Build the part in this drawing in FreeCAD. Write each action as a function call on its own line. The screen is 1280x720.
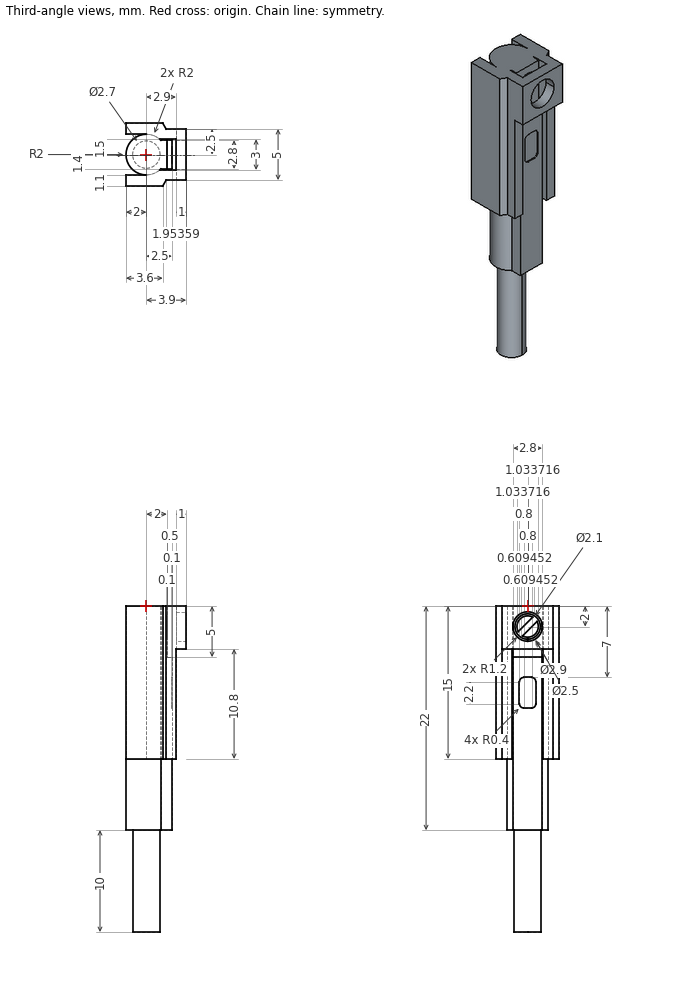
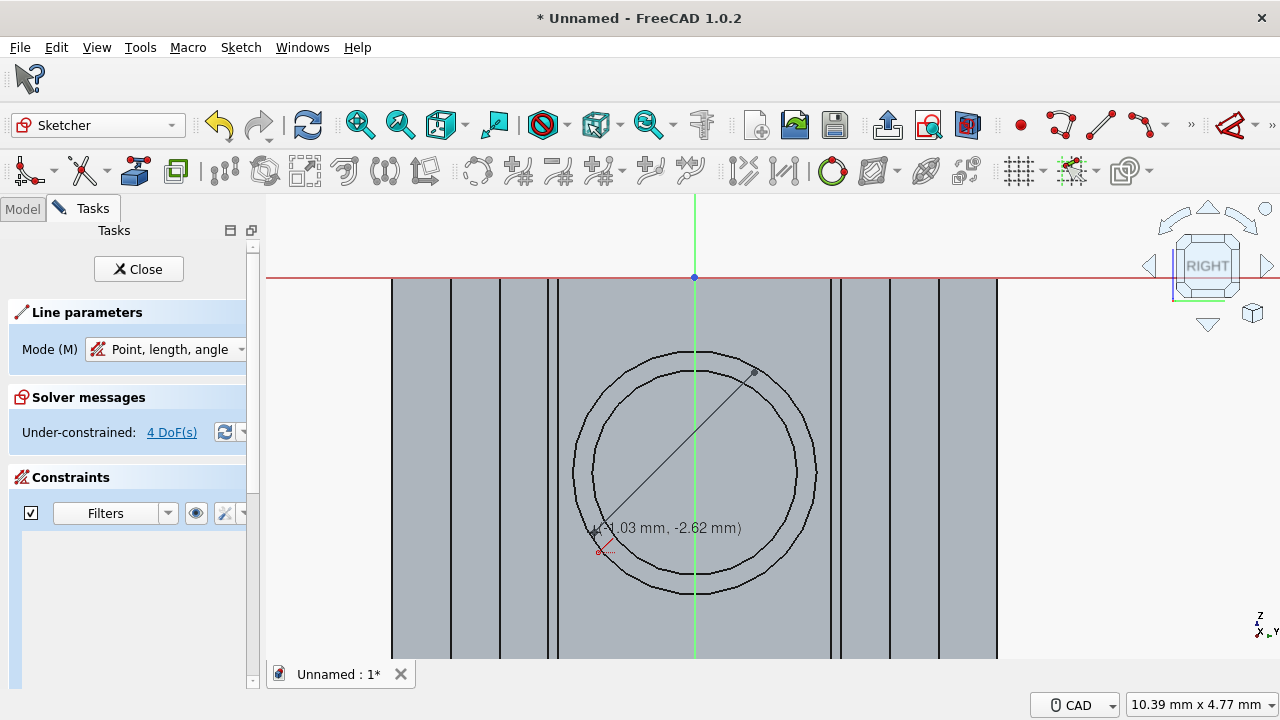
click(635, 574)
click(796, 413)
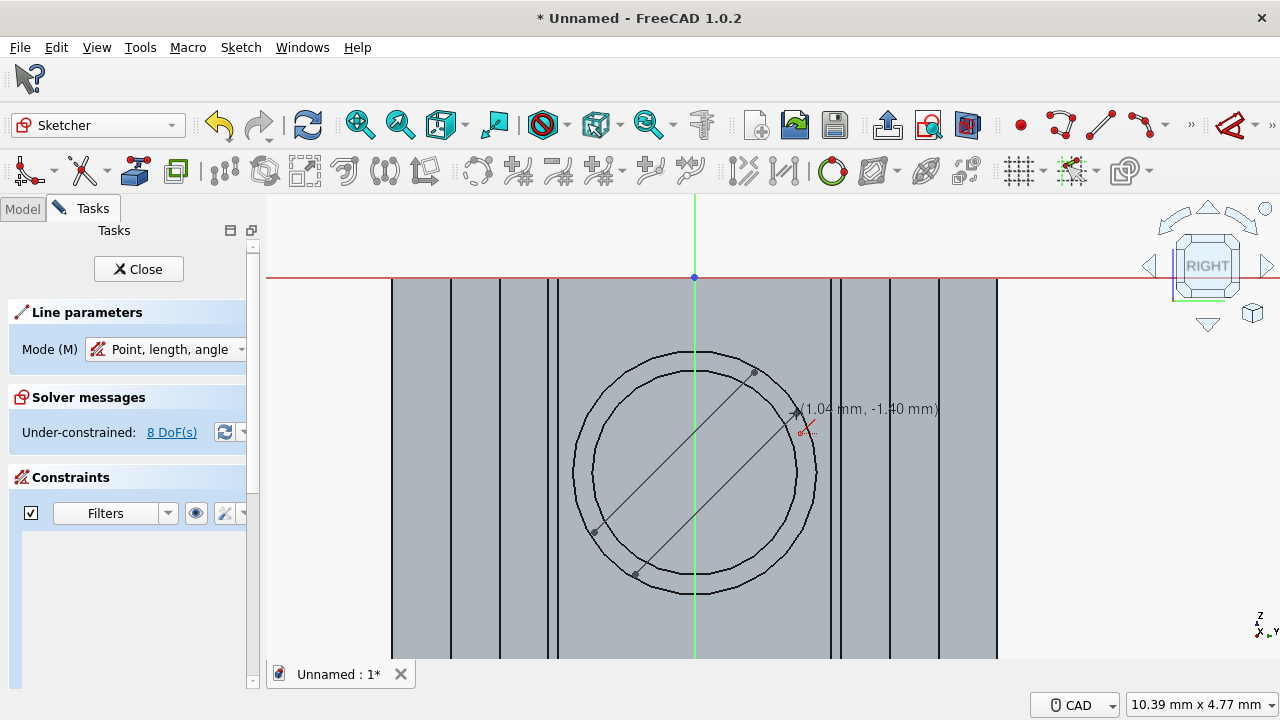
click(1142, 126)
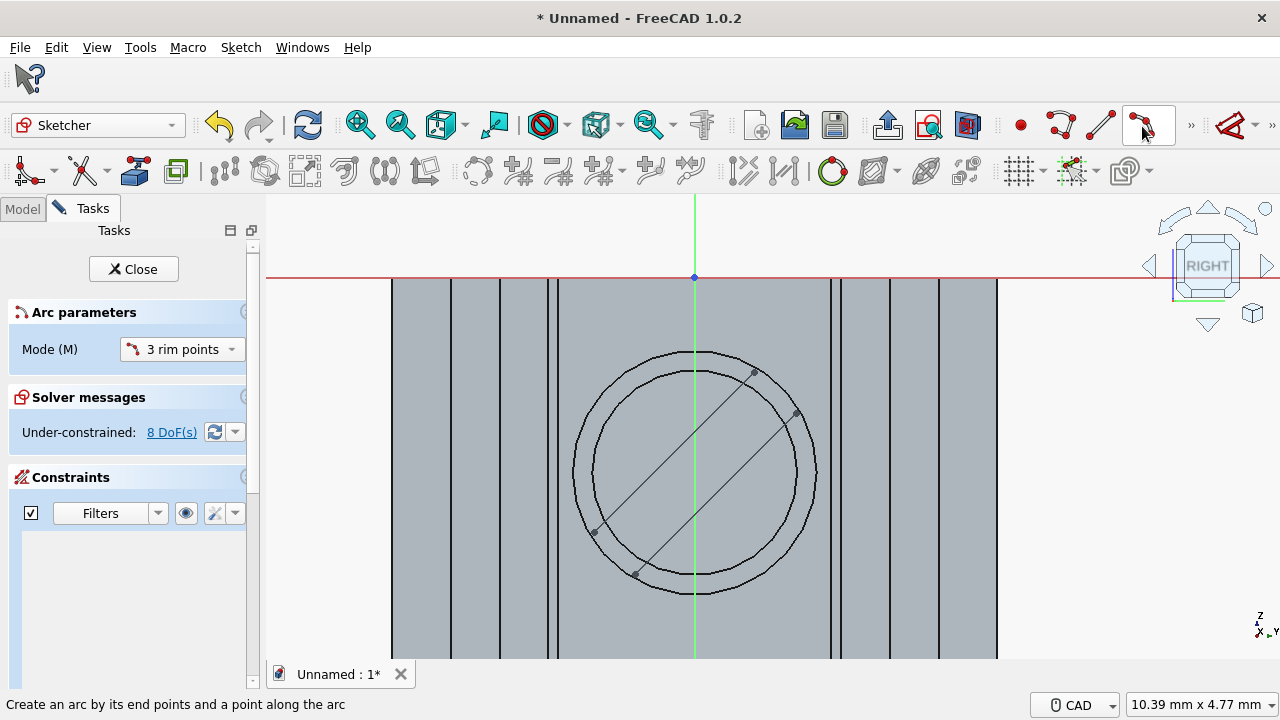
click(594, 533)
click(635, 575)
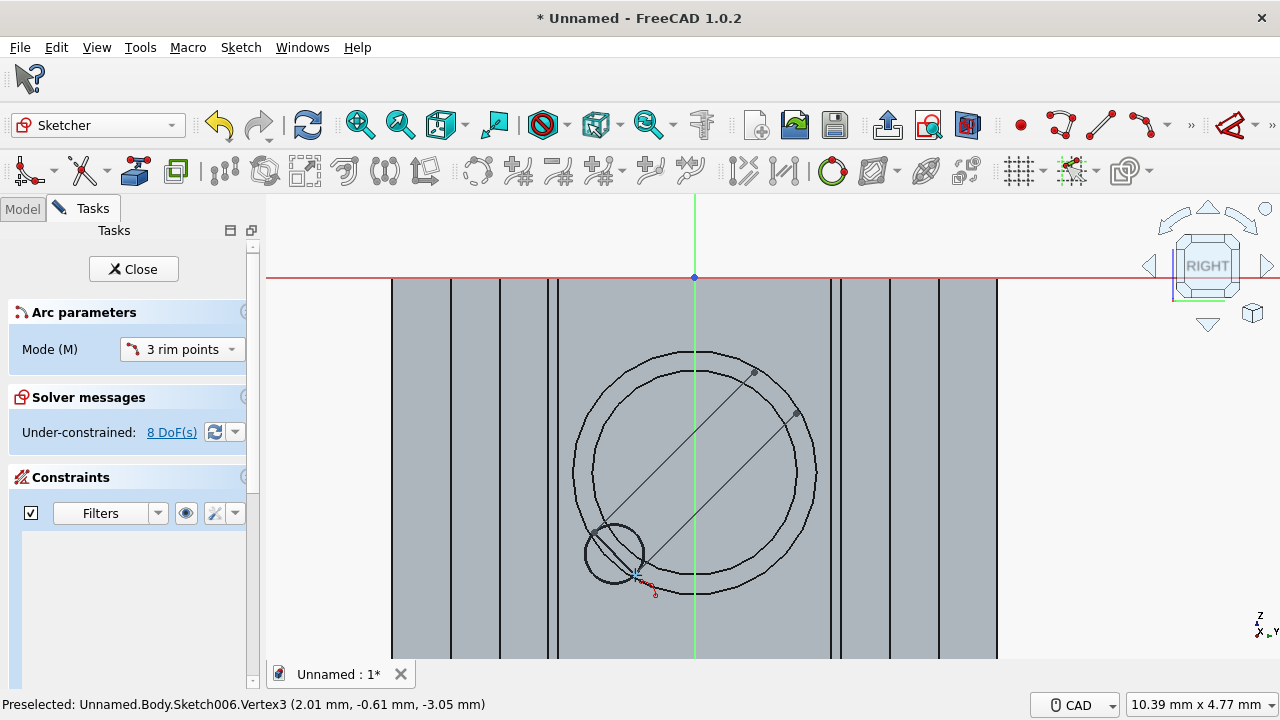
scroll(612, 555, up, 8)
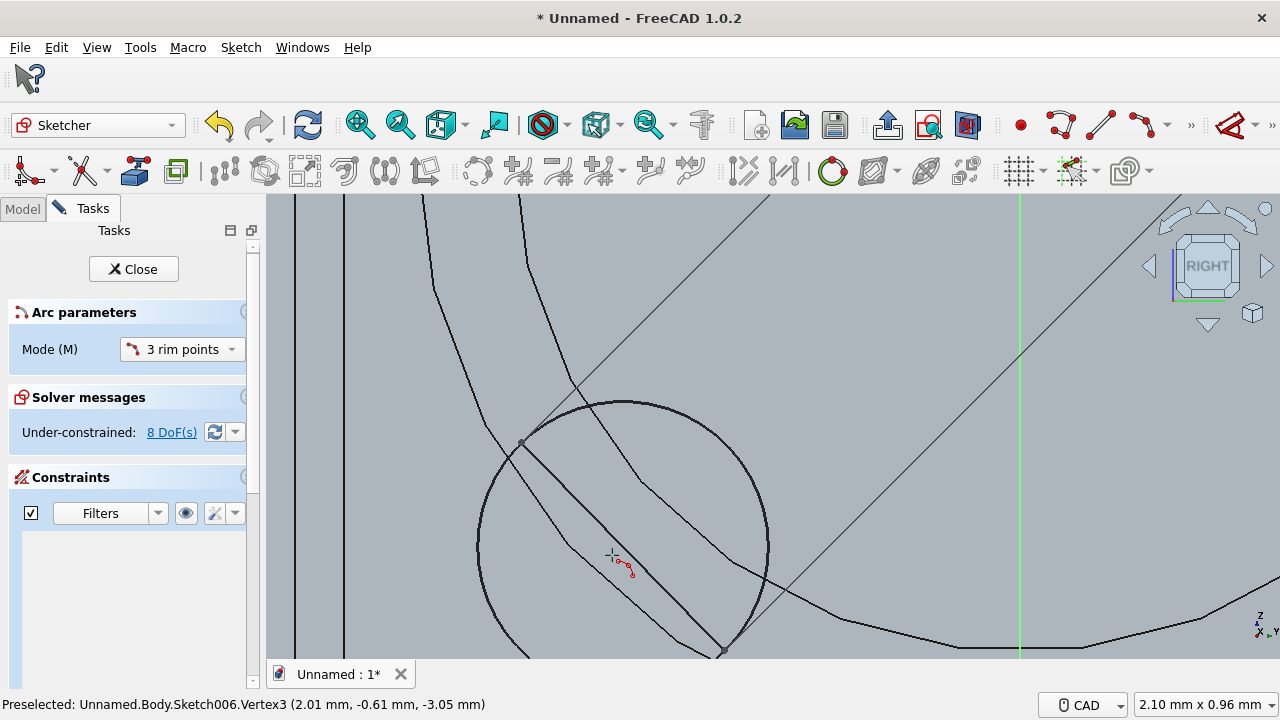
click(610, 554)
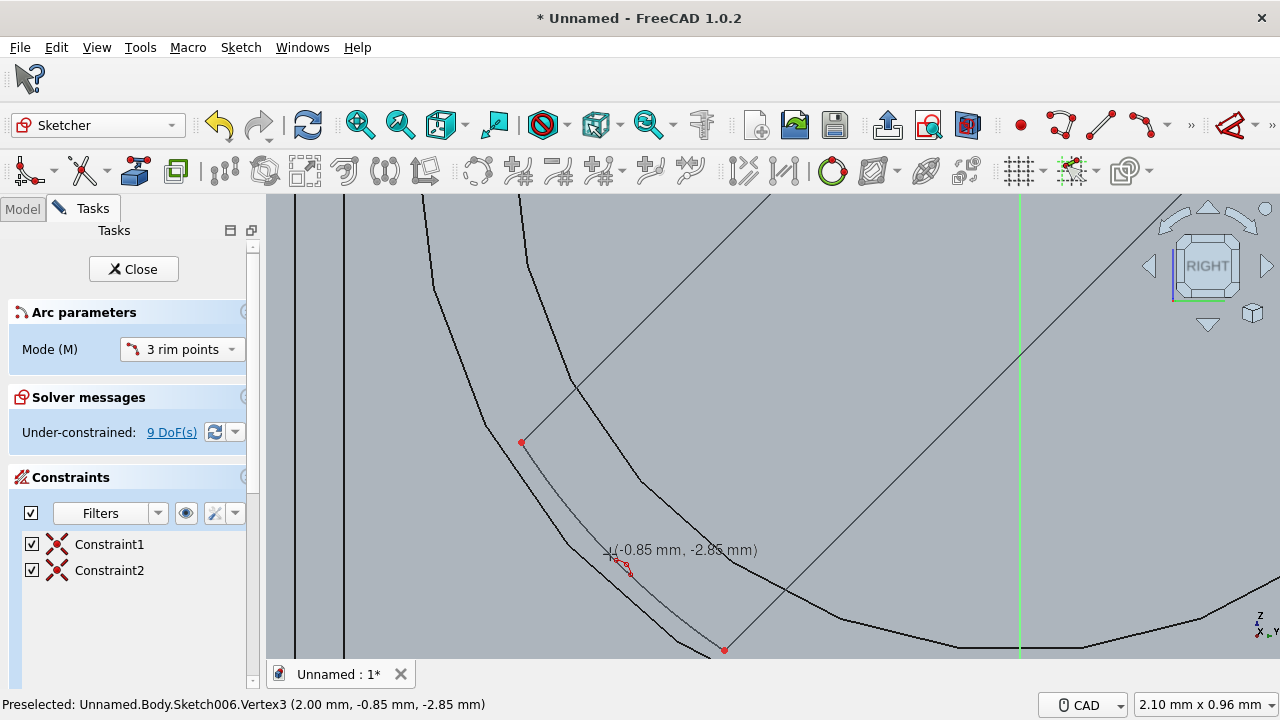
scroll(625, 557, down, 8)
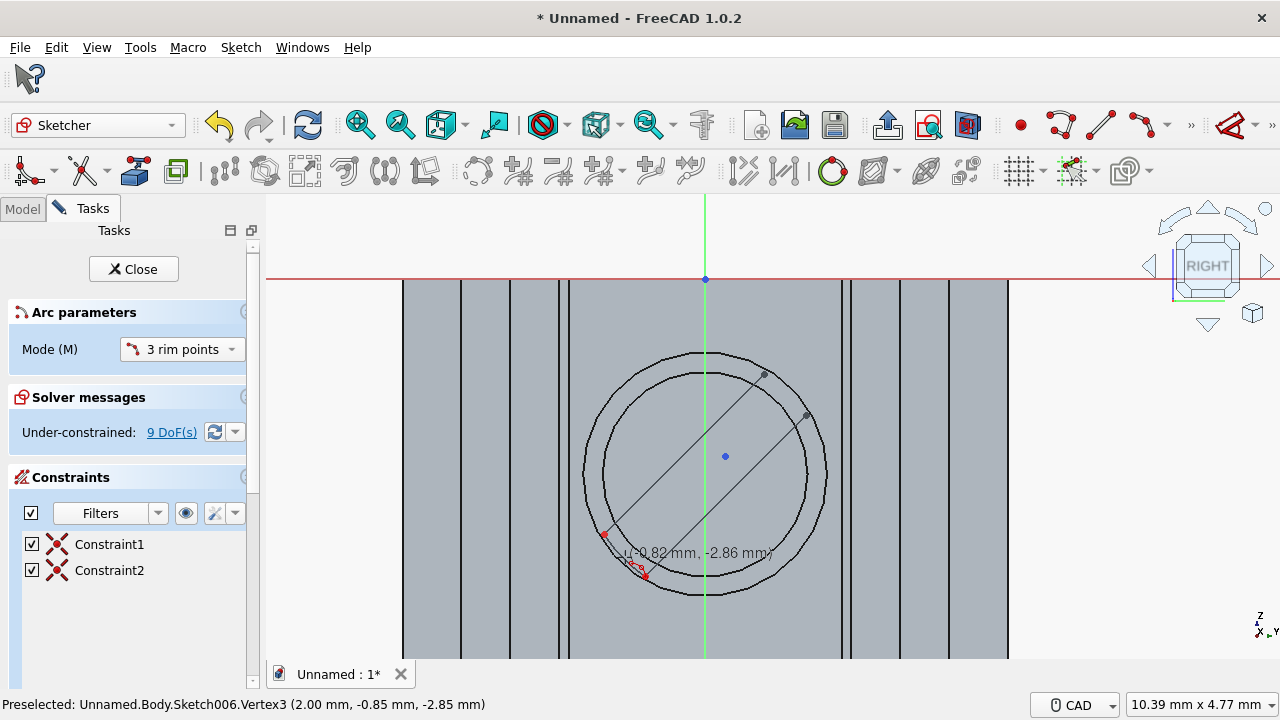
click(806, 416)
click(764, 375)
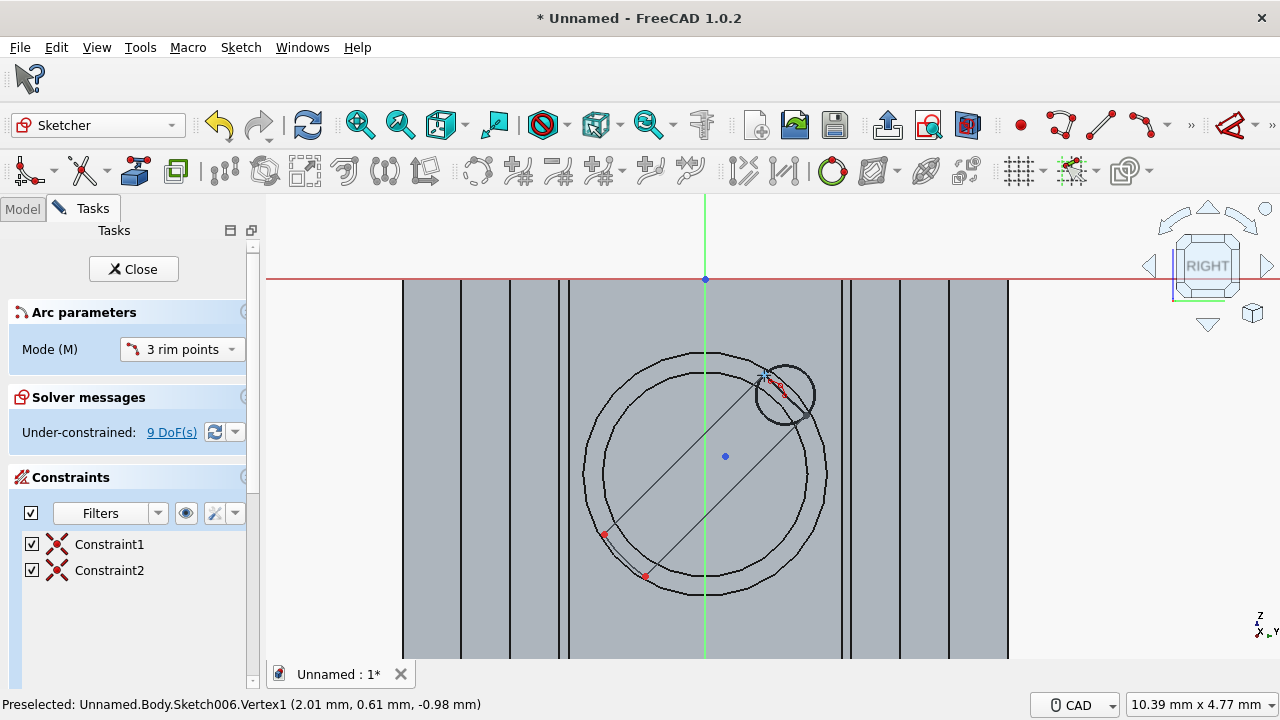
scroll(788, 392, up, 8)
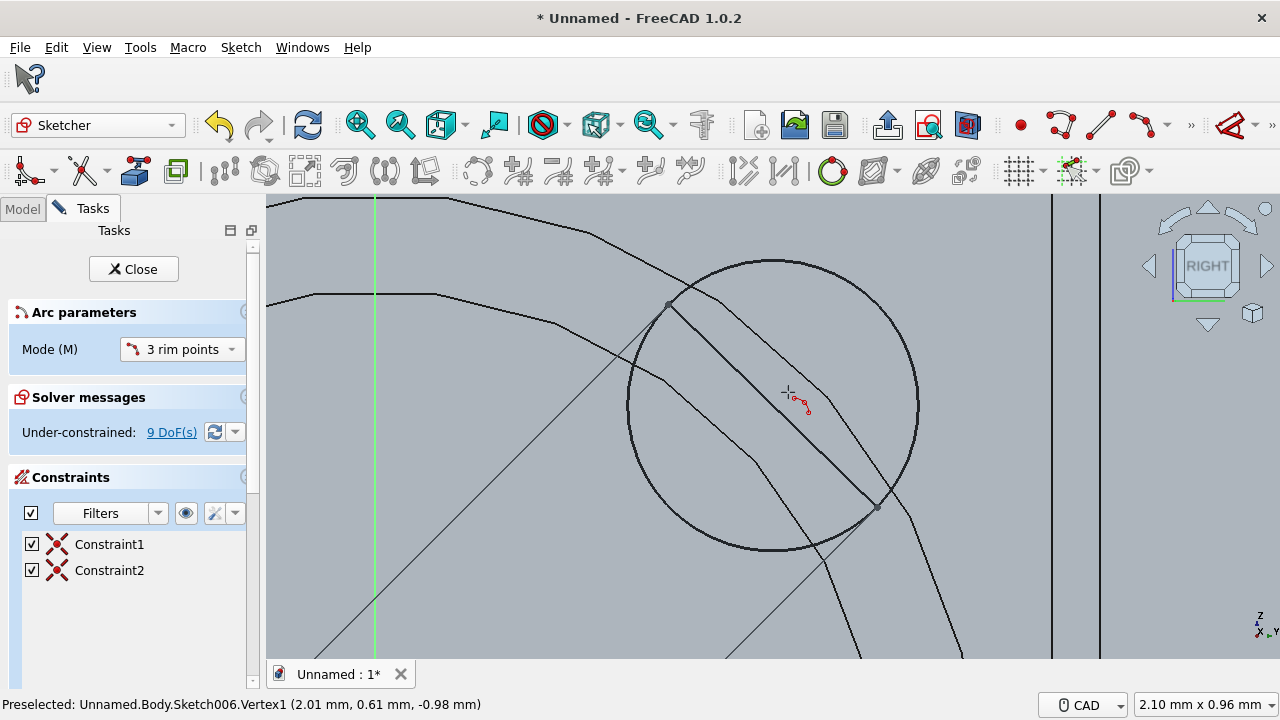
click(785, 388)
key(Escape)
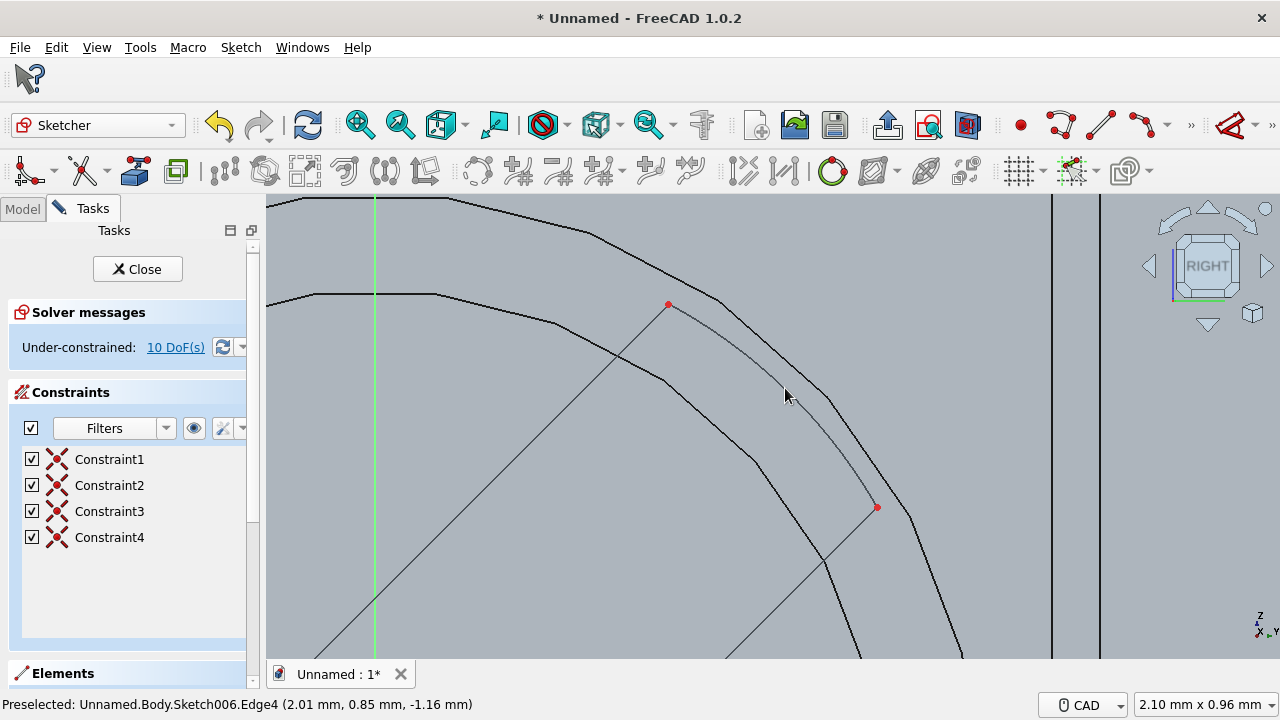
scroll(788, 392, down, 8)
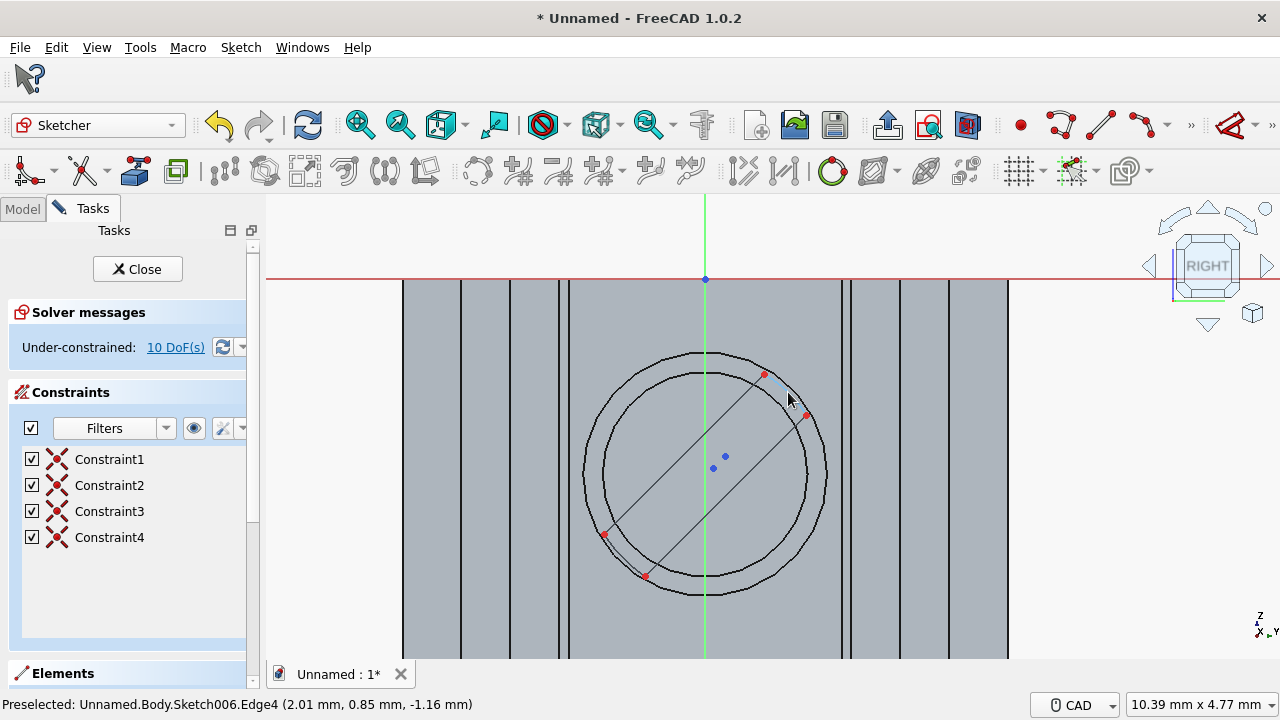
click(615, 549)